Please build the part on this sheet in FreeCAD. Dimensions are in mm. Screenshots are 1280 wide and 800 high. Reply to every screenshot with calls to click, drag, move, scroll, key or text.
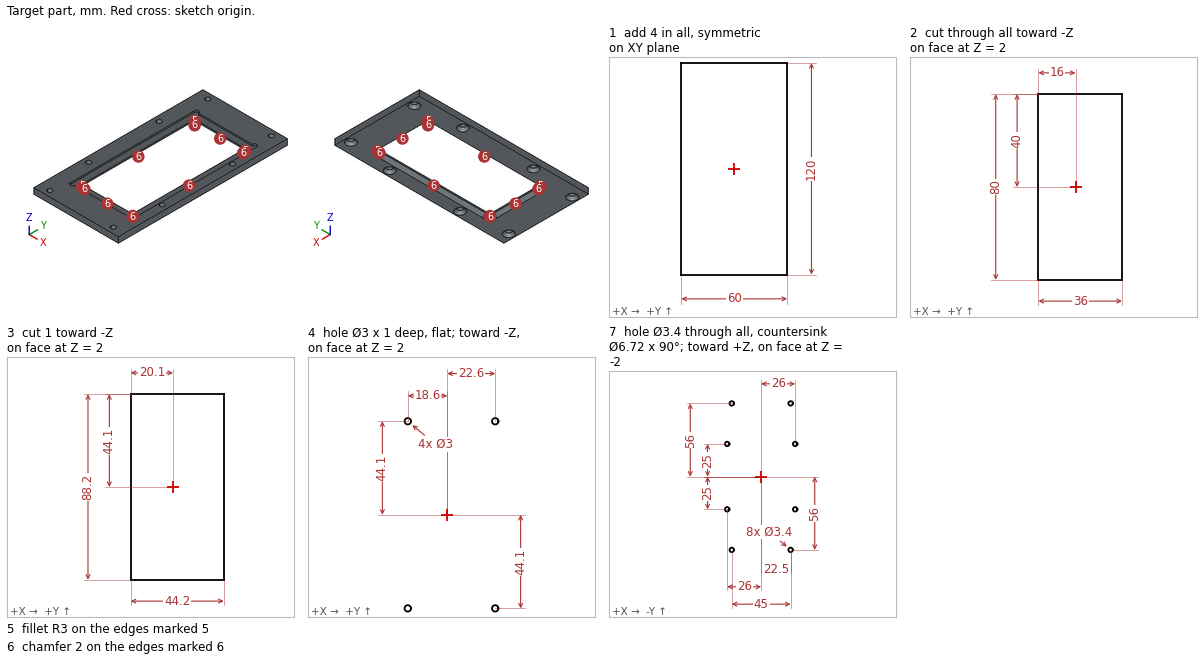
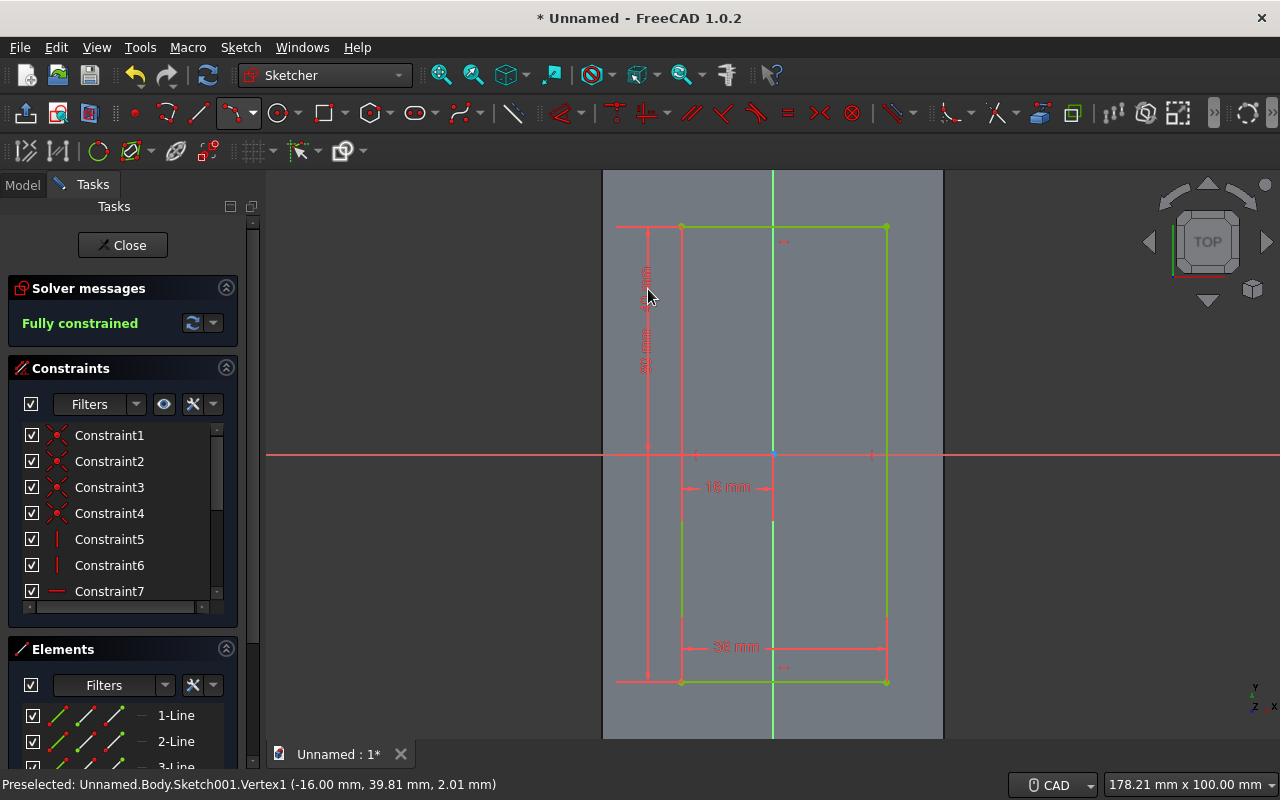
click(123, 245)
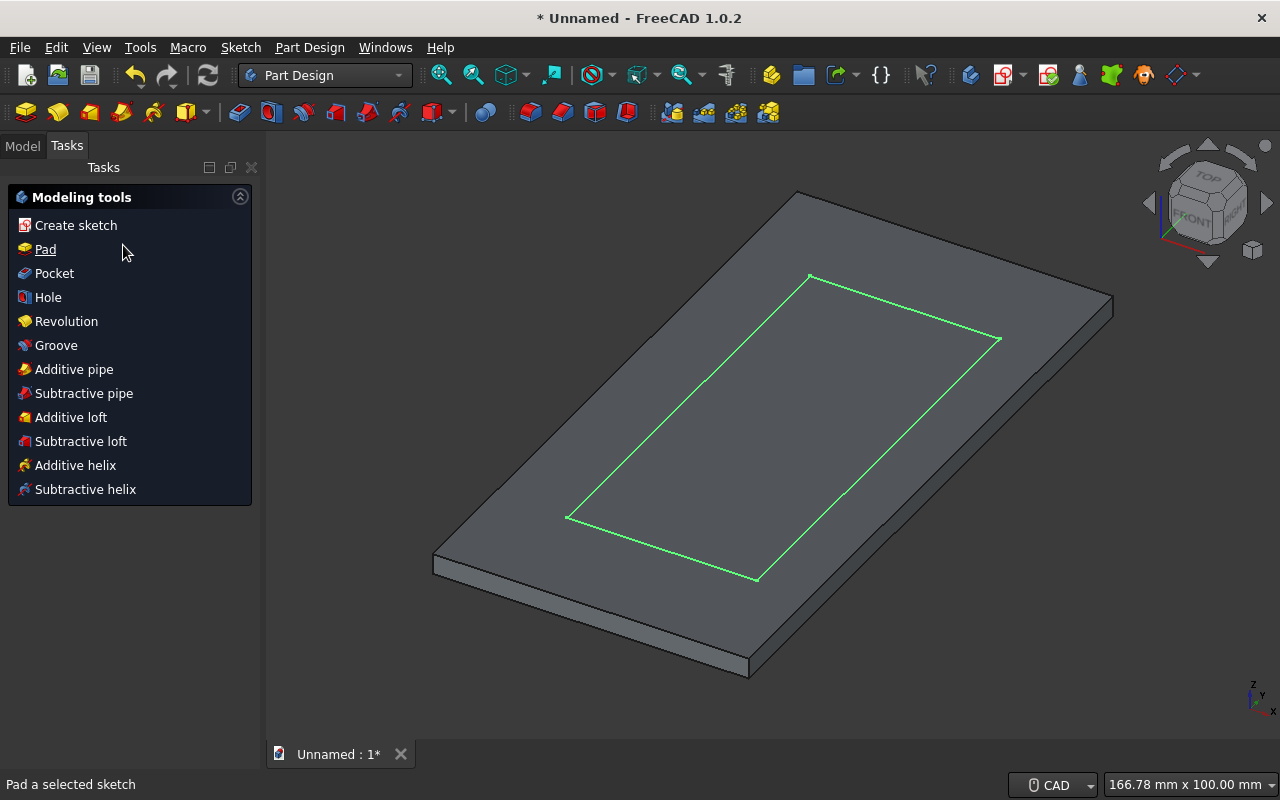
click(240, 112)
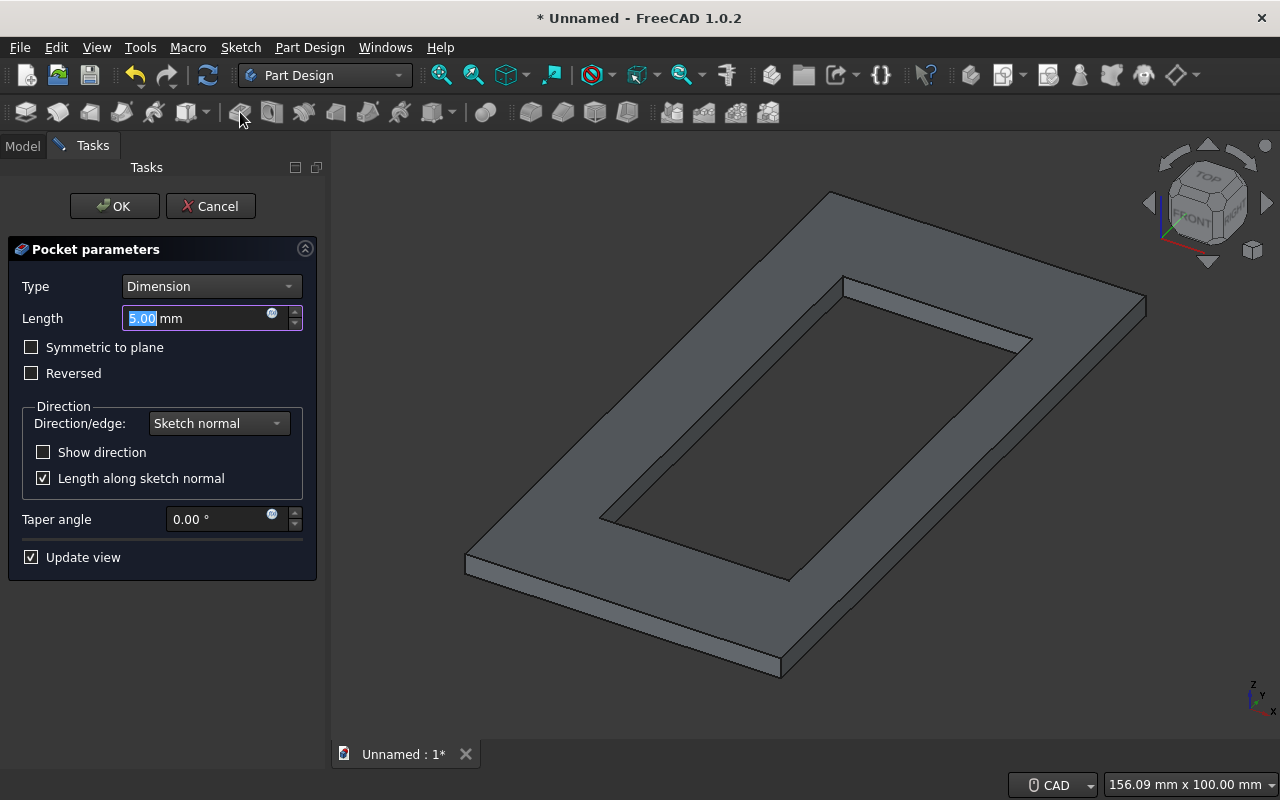
click(212, 286)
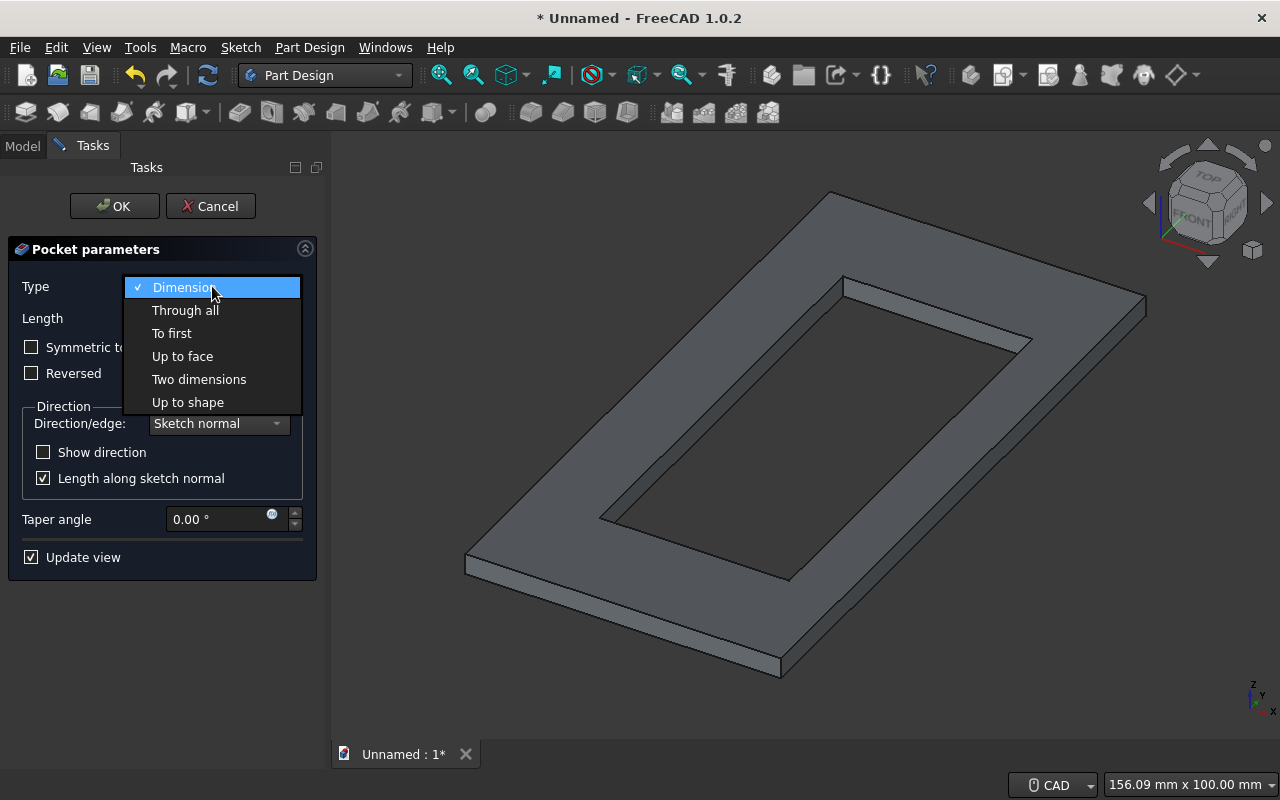
click(212, 310)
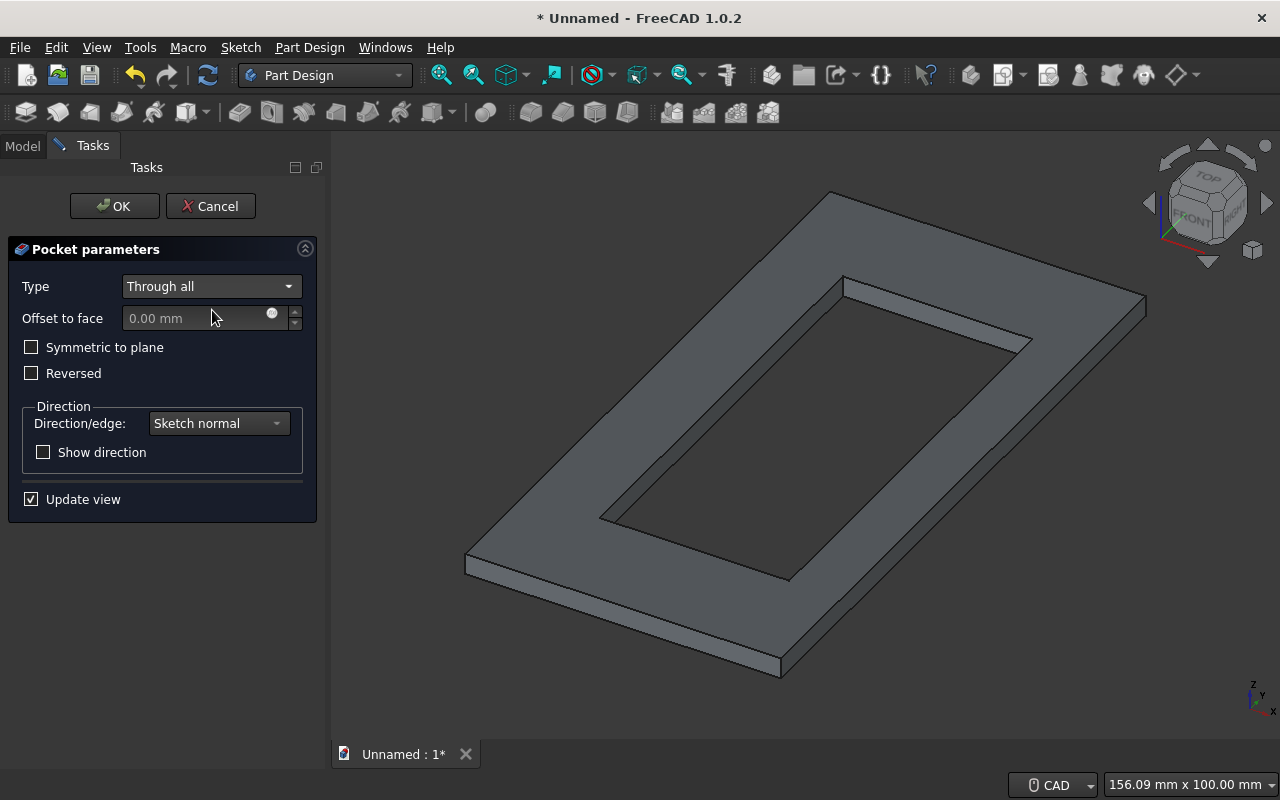
click(115, 206)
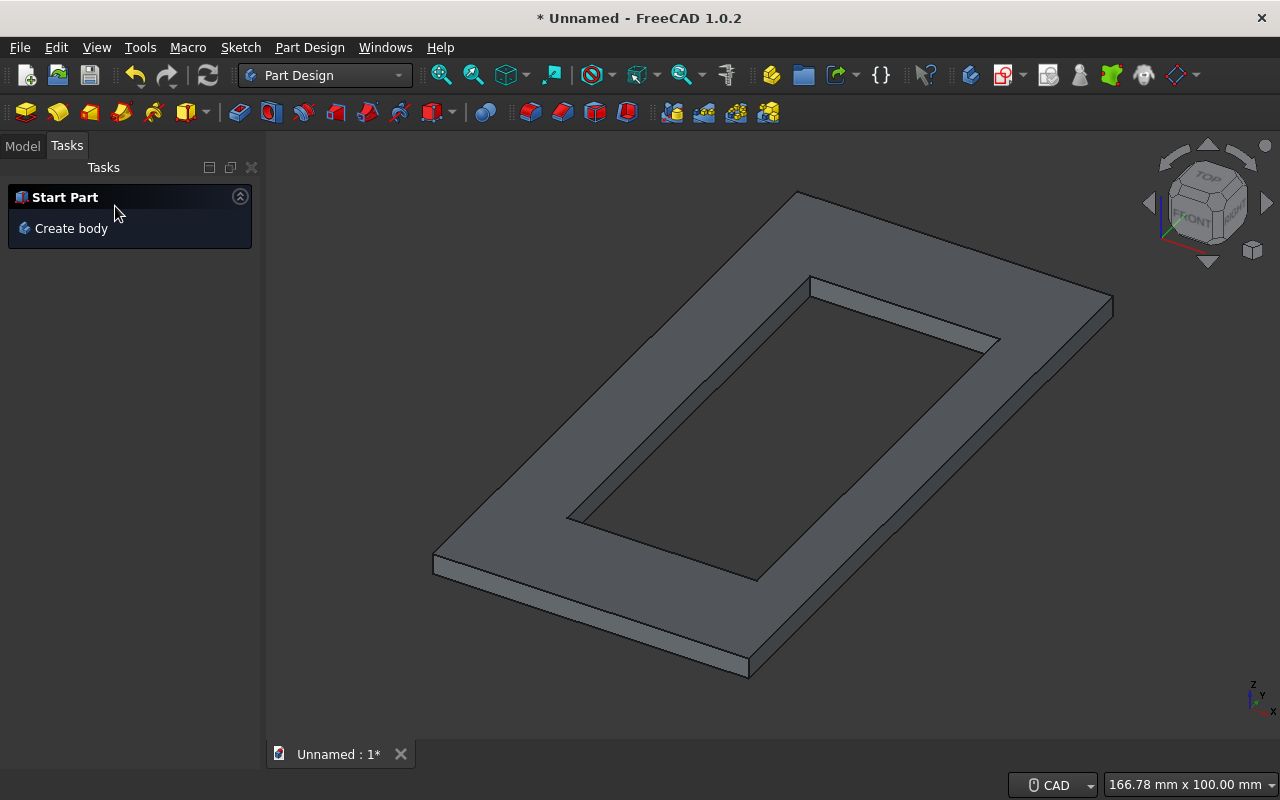
click(1020, 299)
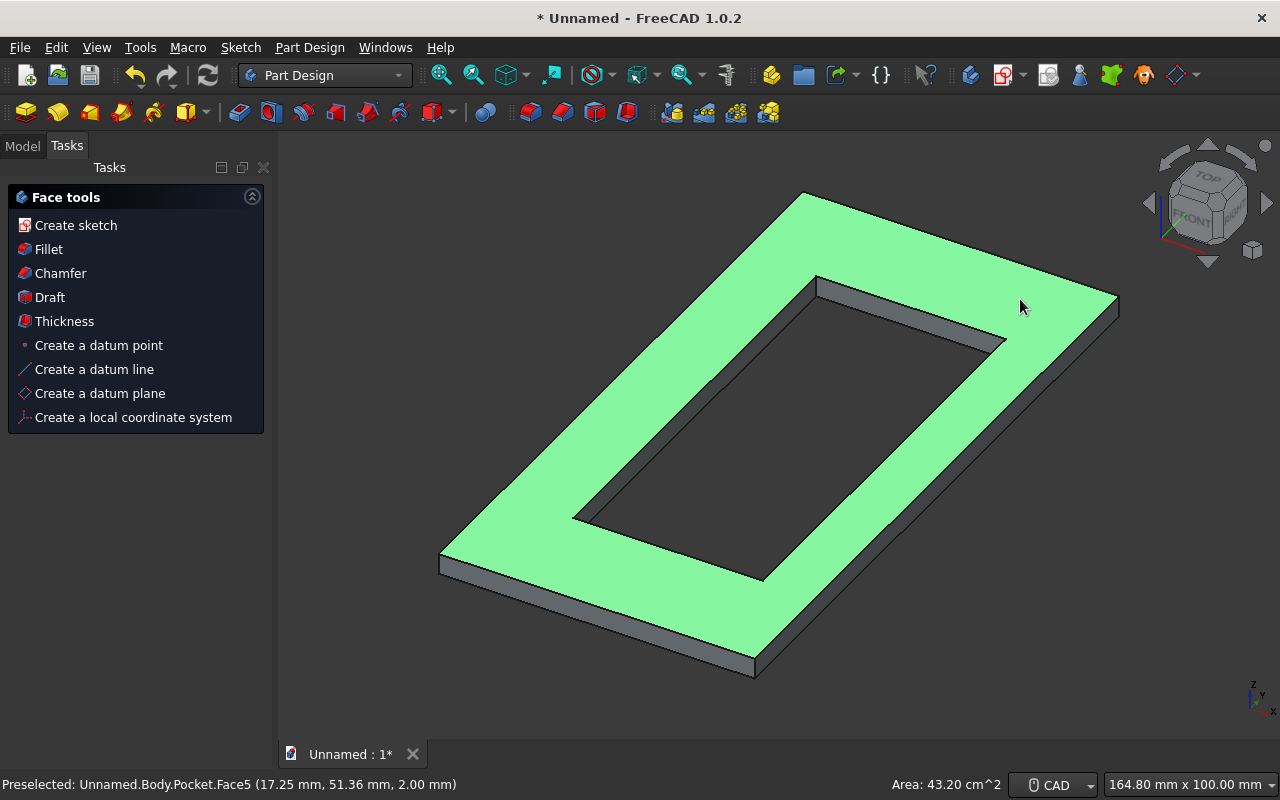
click(1004, 76)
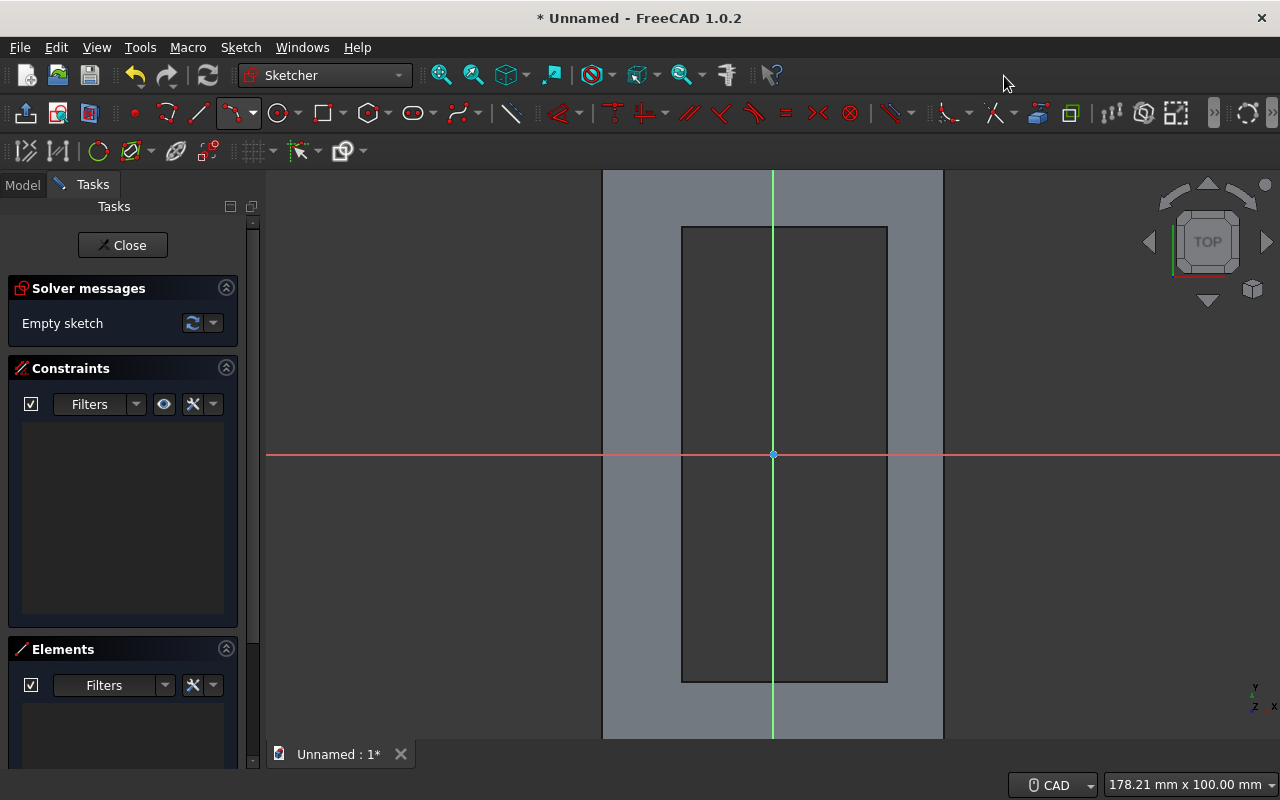
scroll(542, 455, down, 2)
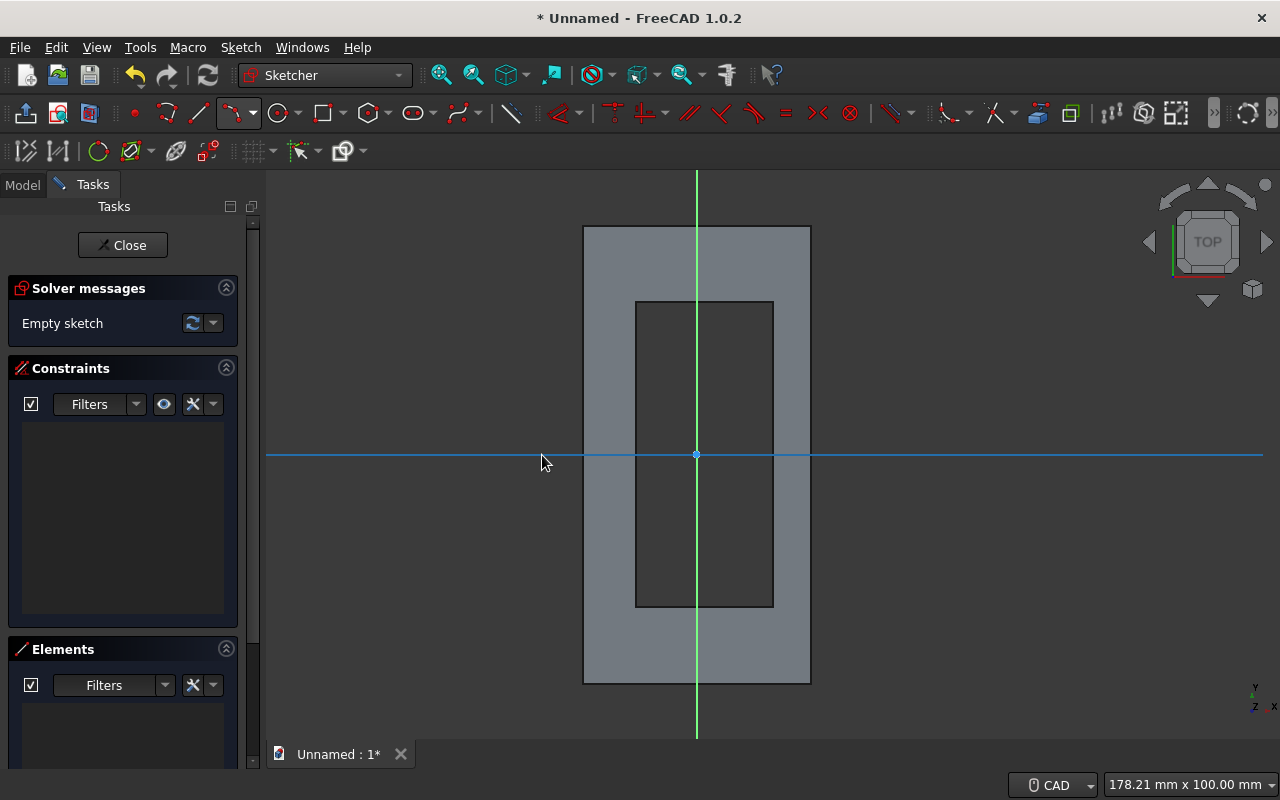
click(324, 114)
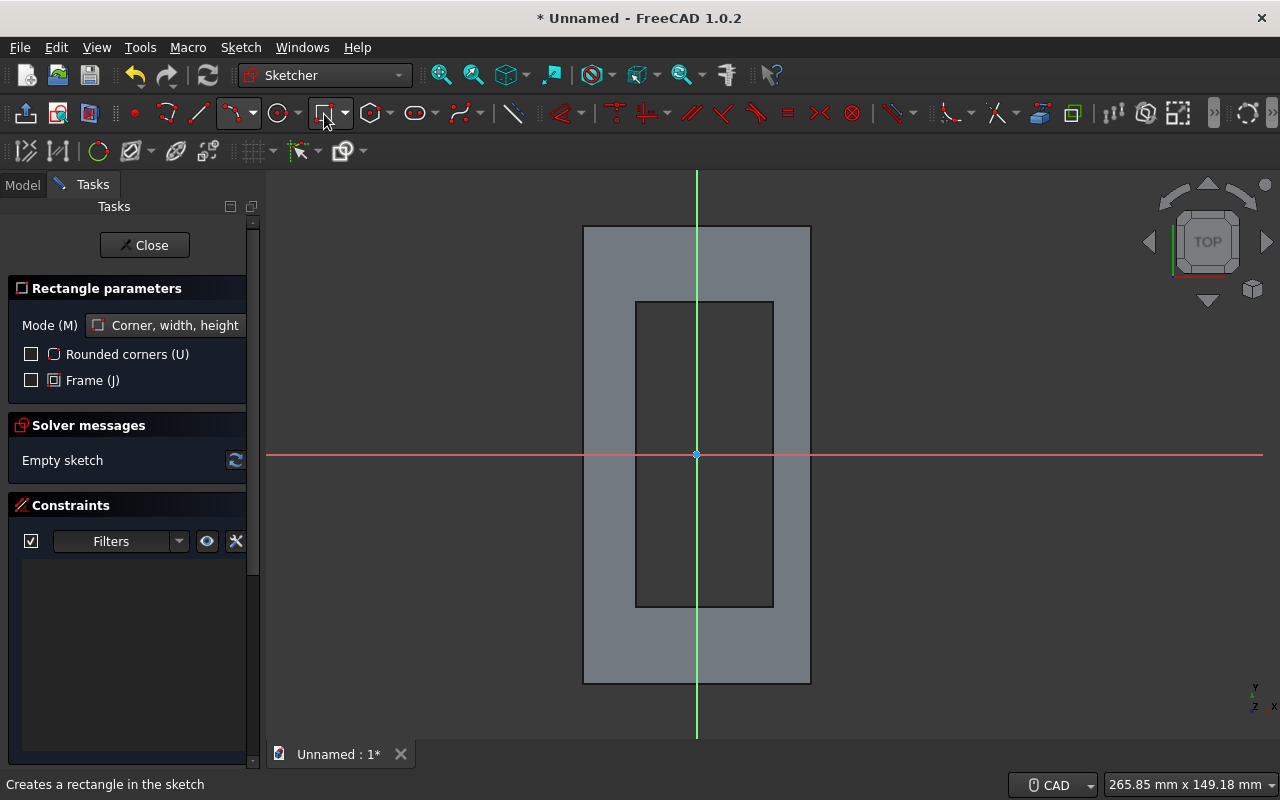
click(620, 287)
click(789, 623)
key(Escape)